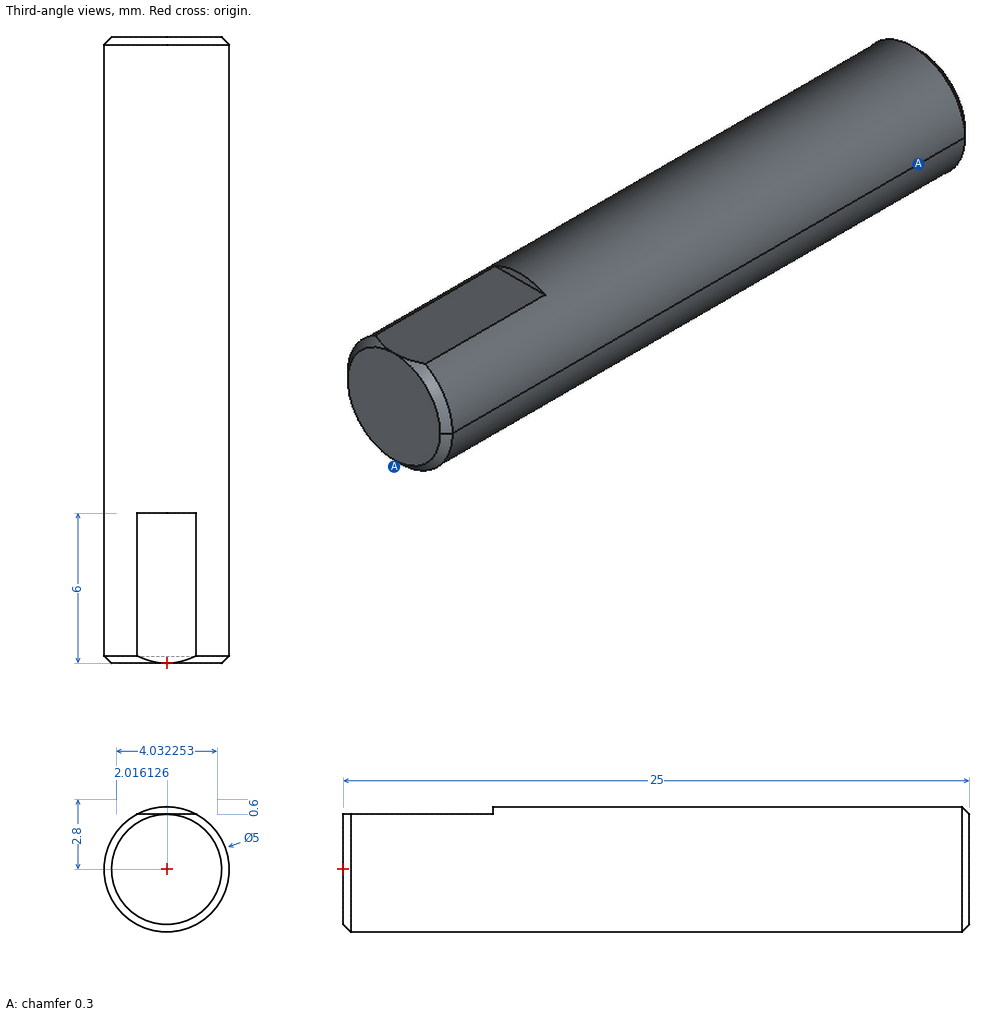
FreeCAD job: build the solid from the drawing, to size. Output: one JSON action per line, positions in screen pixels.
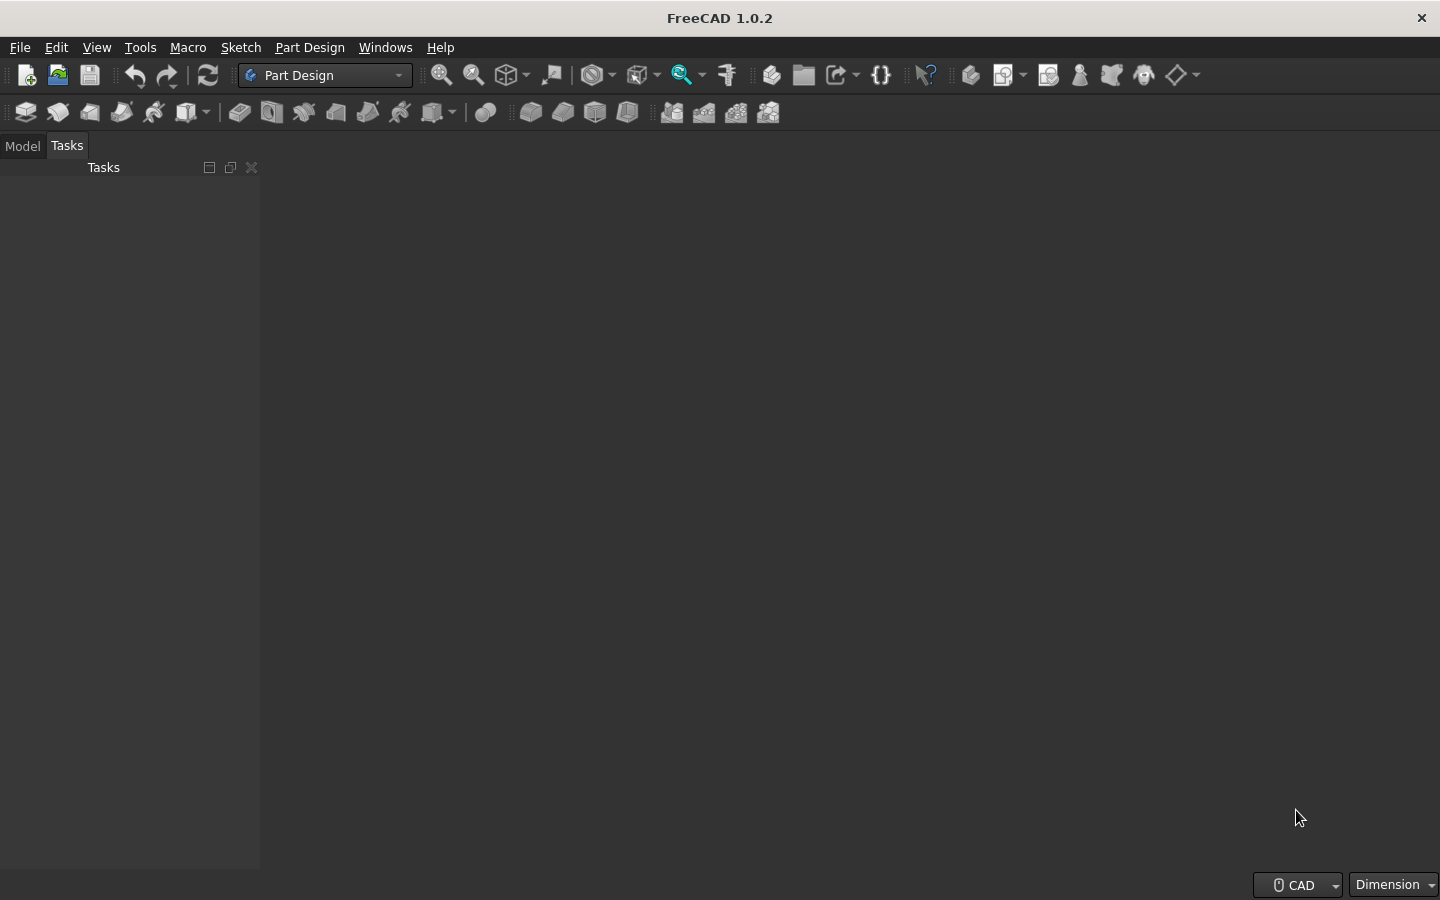
{"action": "left_click", "coordinate": [26, 76]}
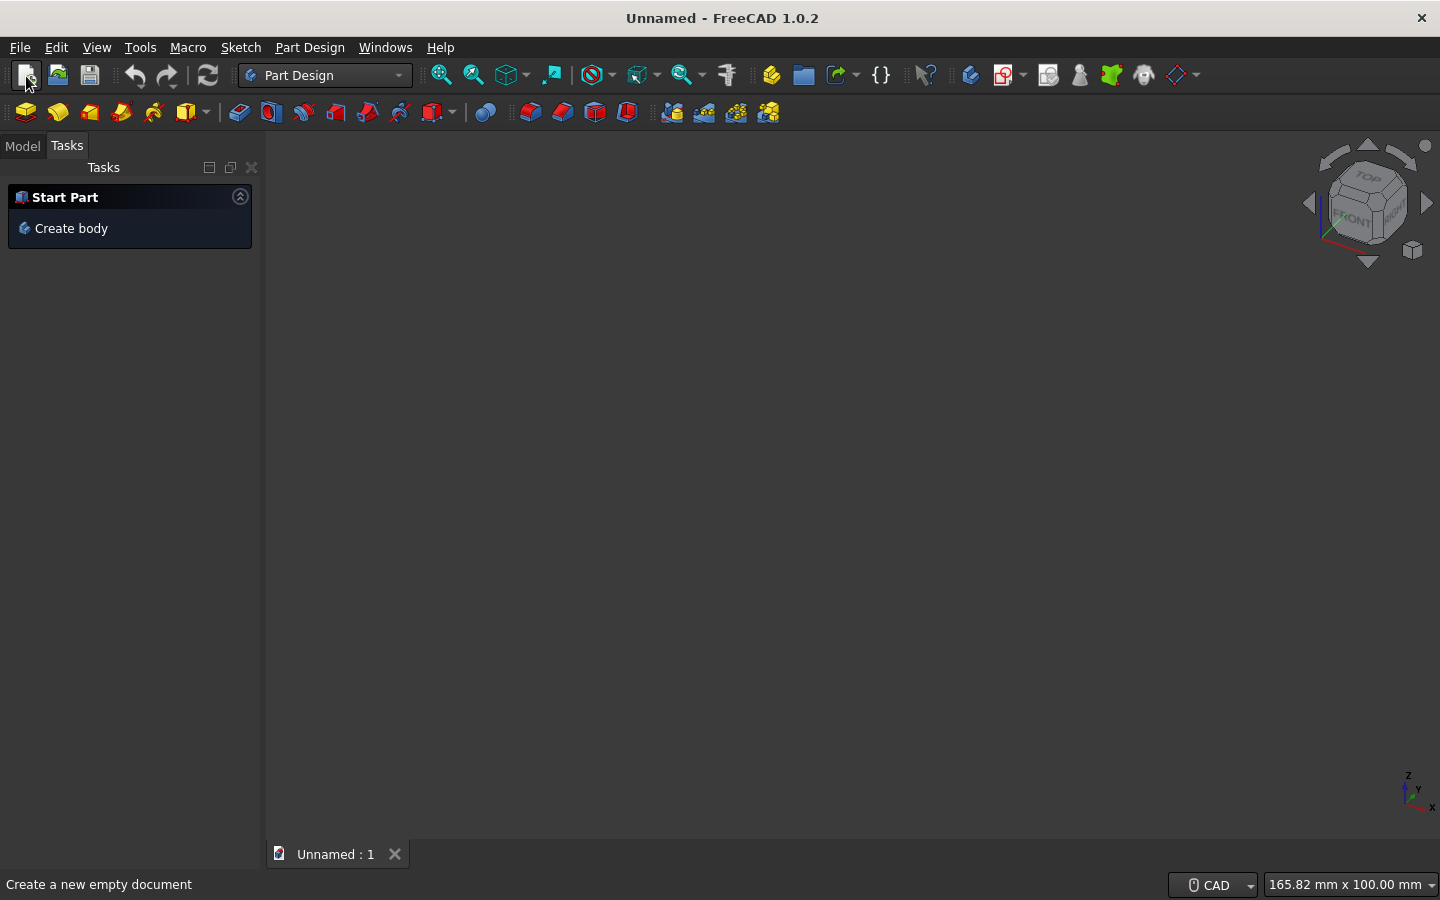
{"action": "left_click", "coordinate": [1004, 76]}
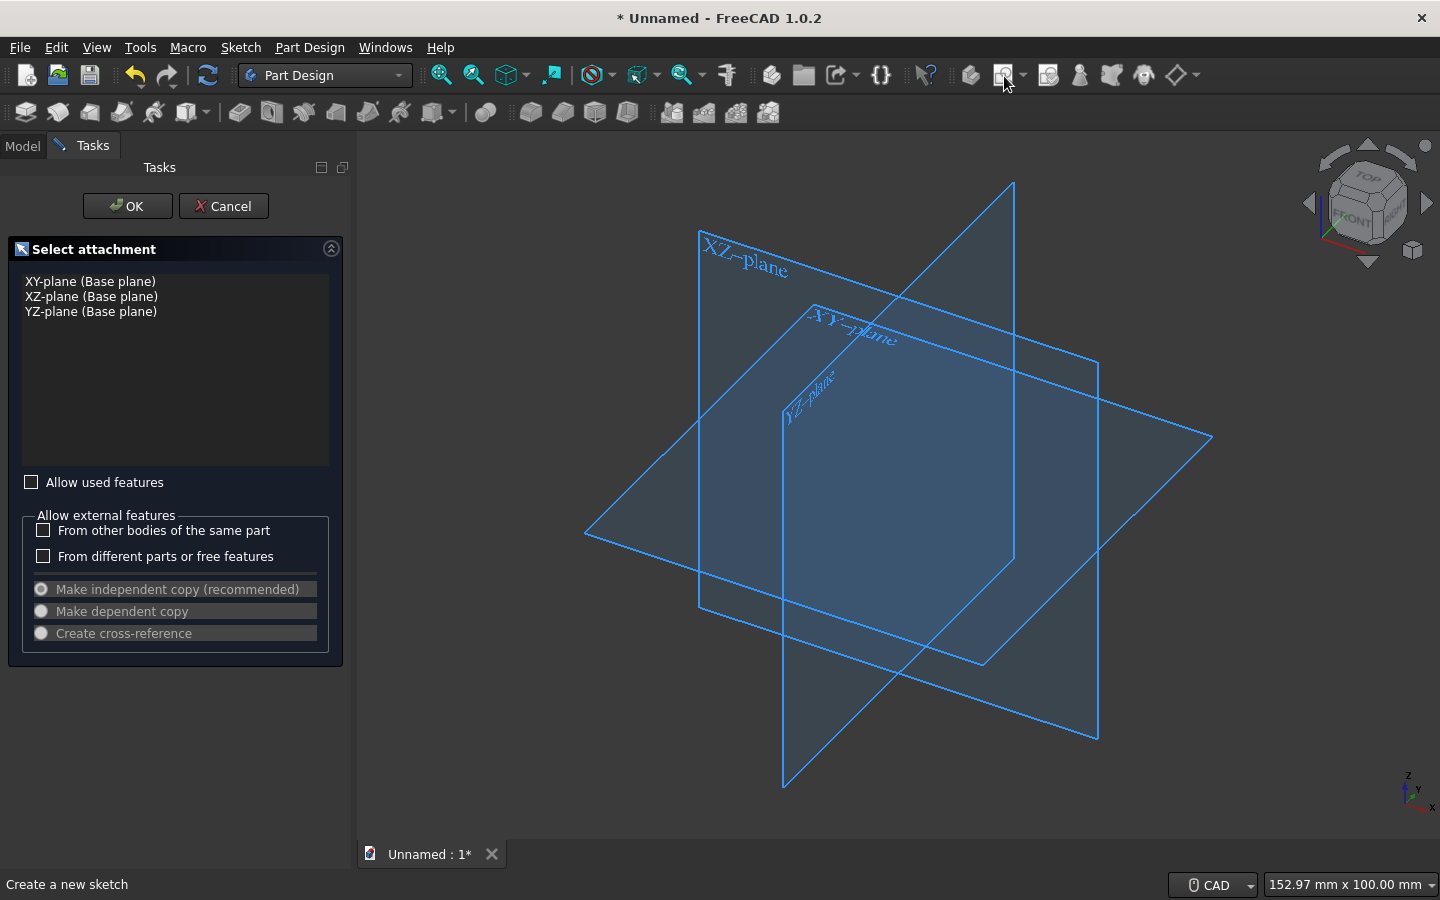
{"action": "left_click", "coordinate": [82, 296]}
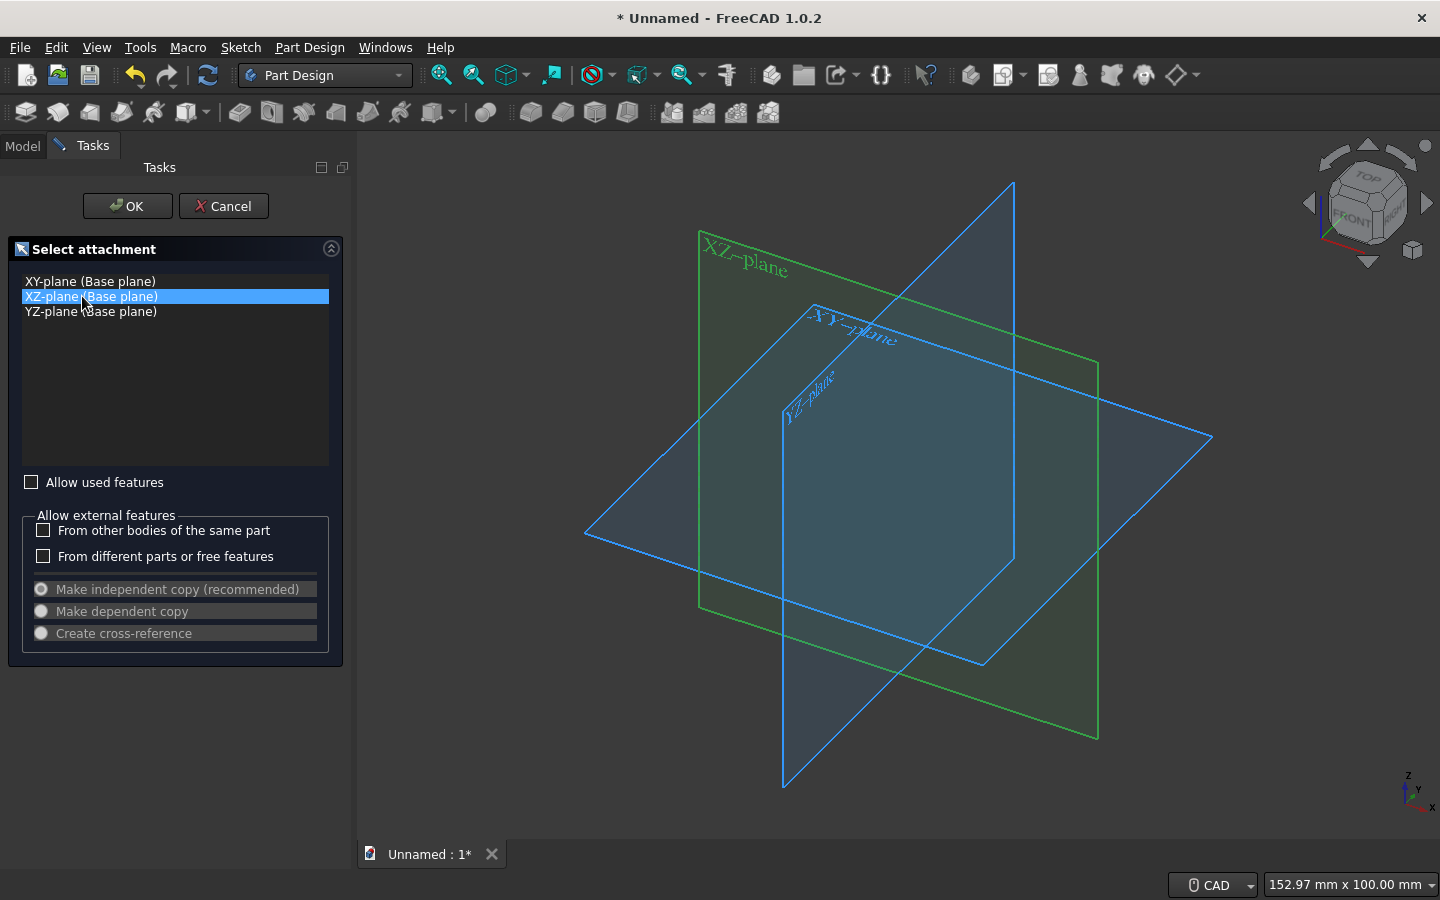
{"action": "left_click", "coordinate": [128, 206]}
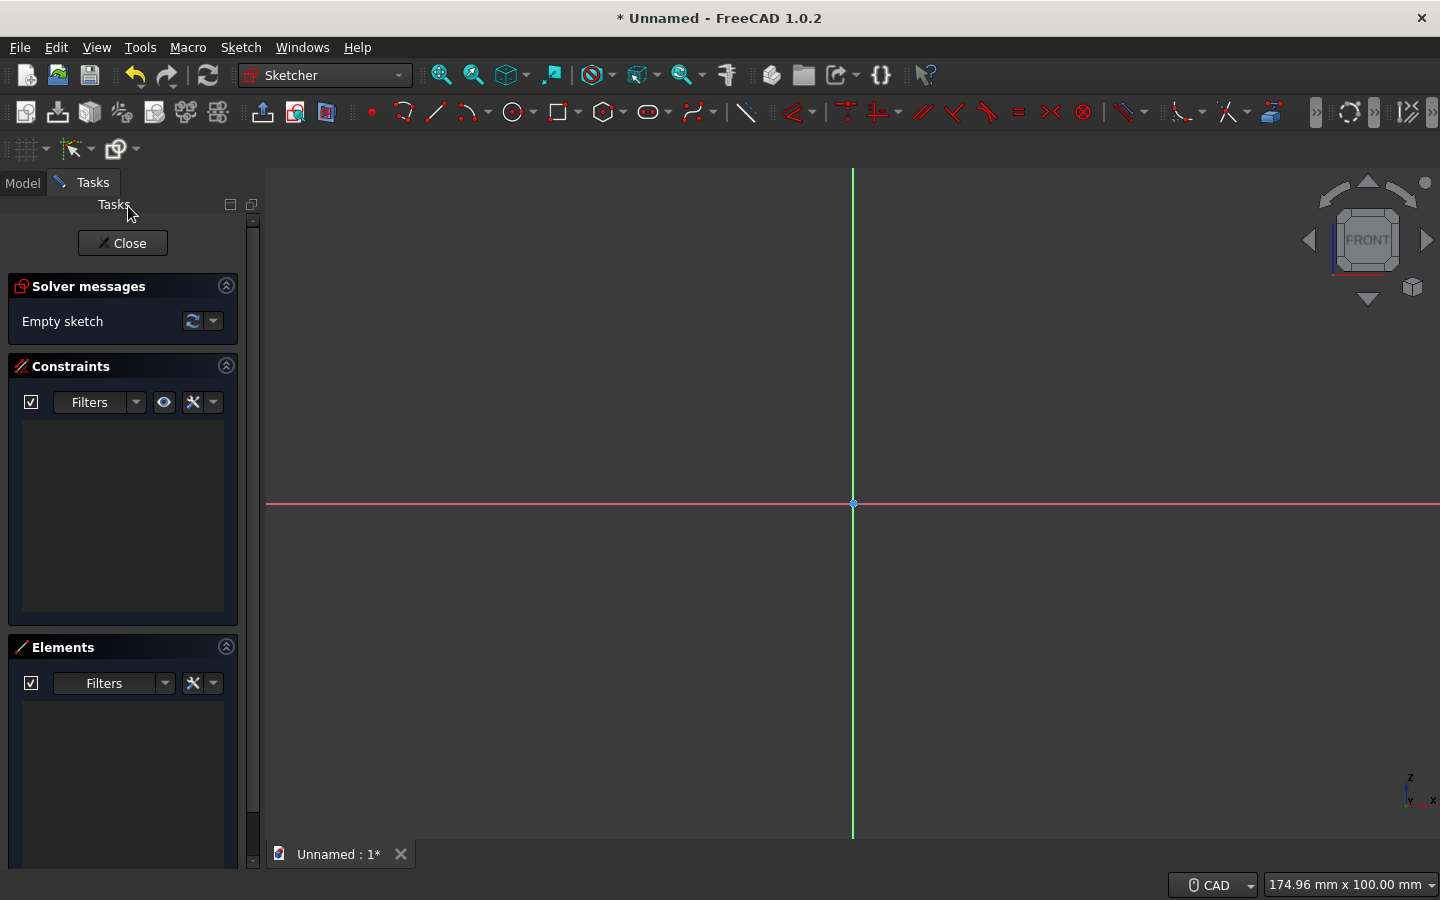
{"action": "scroll", "coordinate": [858, 504], "scroll_direction": "up", "scroll_amount": 13}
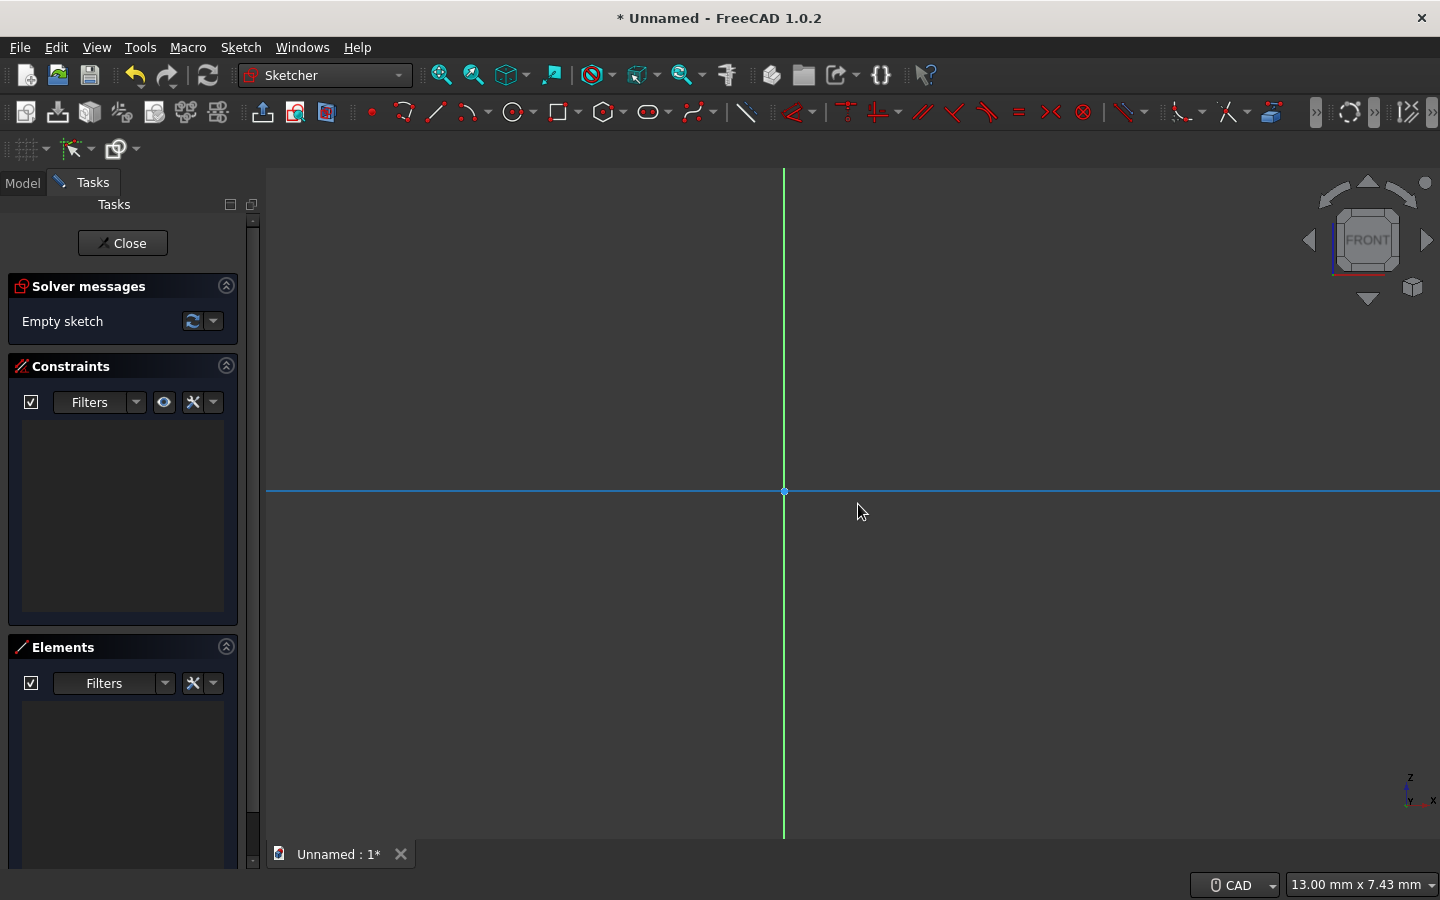
{"action": "left_click", "coordinate": [514, 112]}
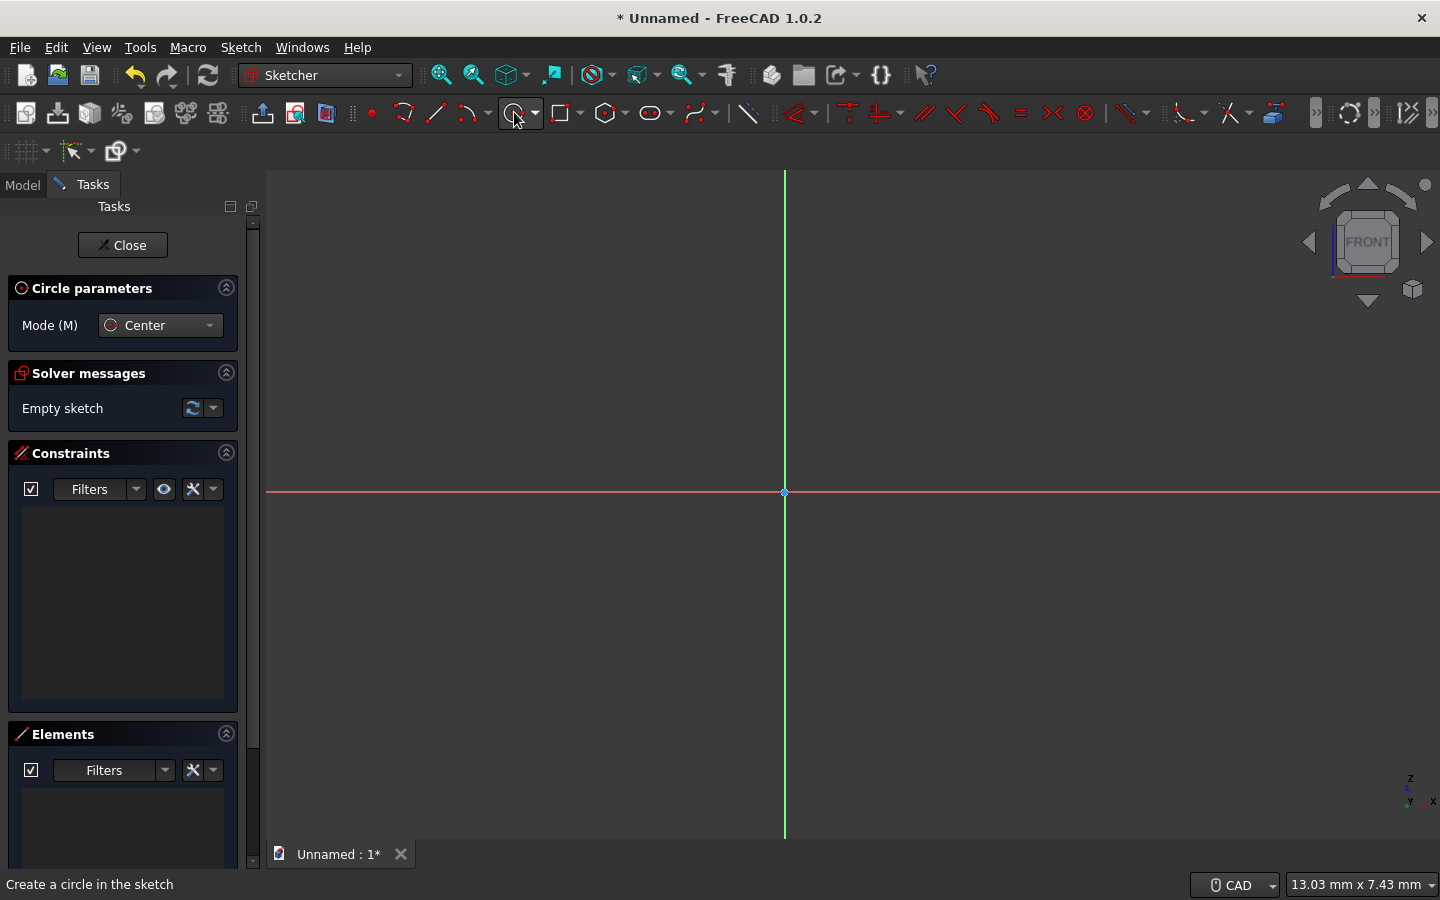
{"action": "left_click", "coordinate": [785, 492]}
{"action": "mouse_move", "coordinate": [944, 333]}